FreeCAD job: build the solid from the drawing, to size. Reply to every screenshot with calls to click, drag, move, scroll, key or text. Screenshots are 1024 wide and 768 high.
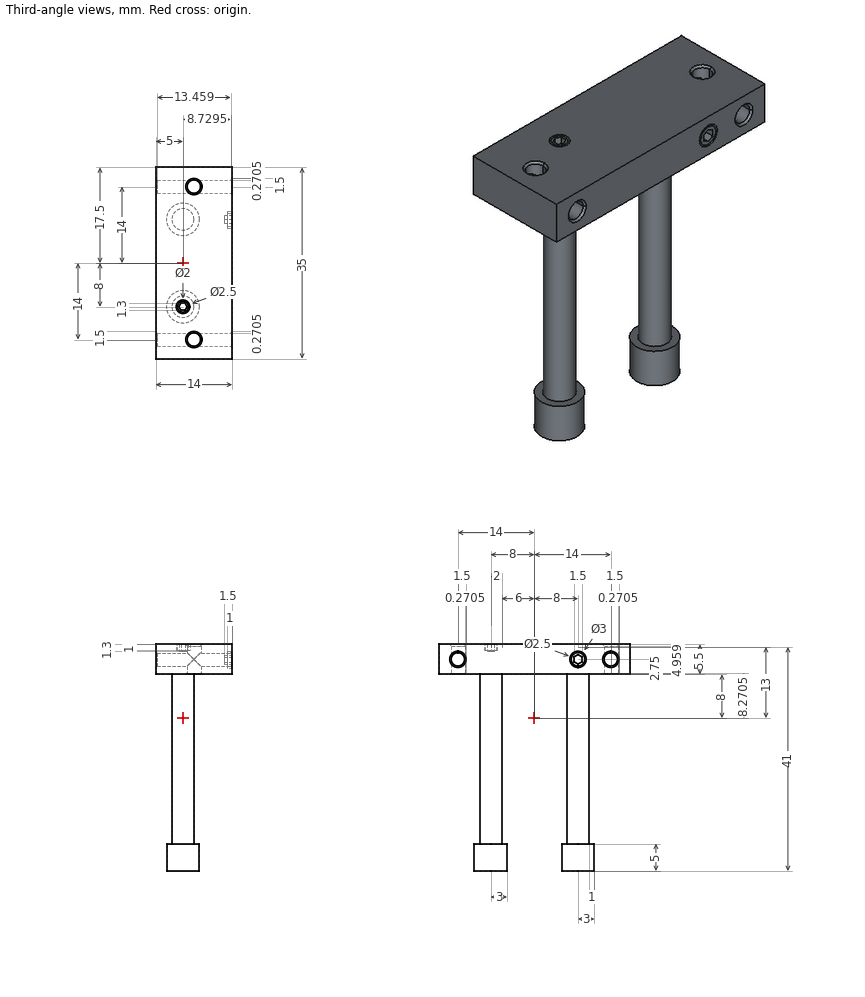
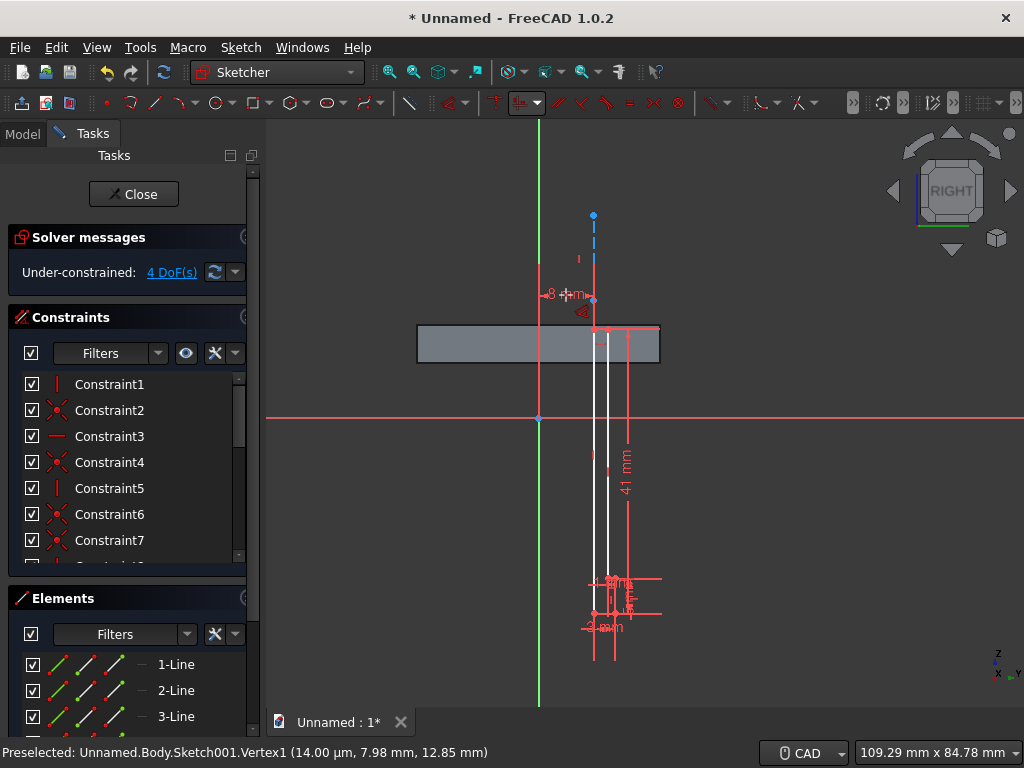
click(594, 301)
click(566, 267)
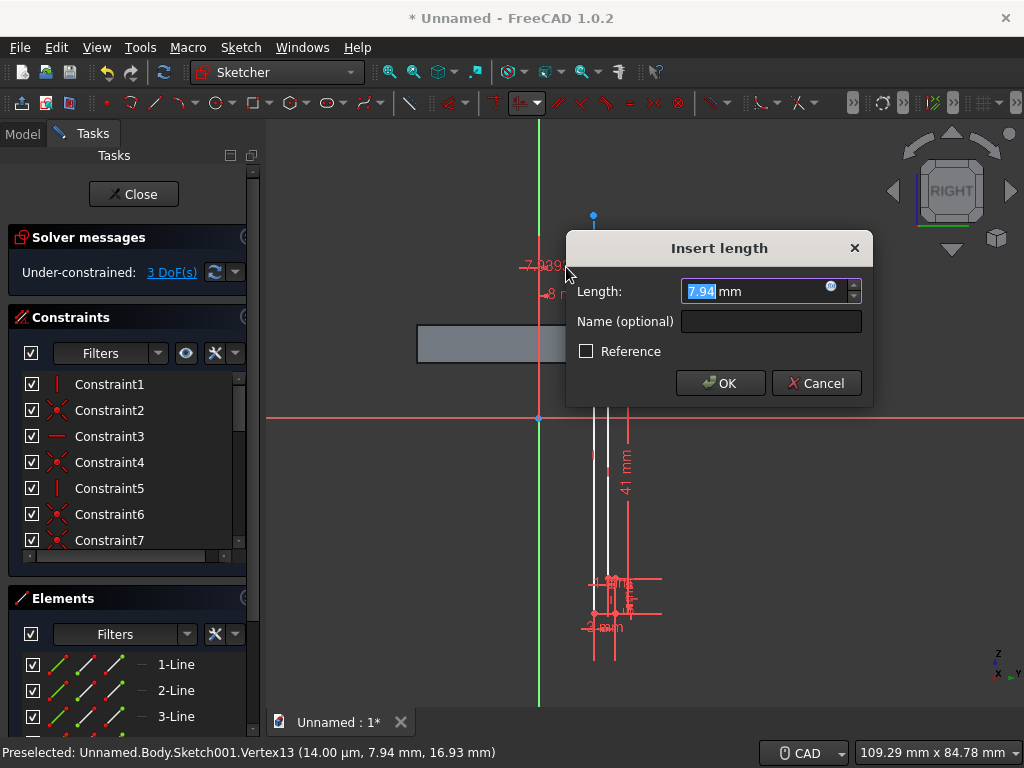
text(8)
key(Return)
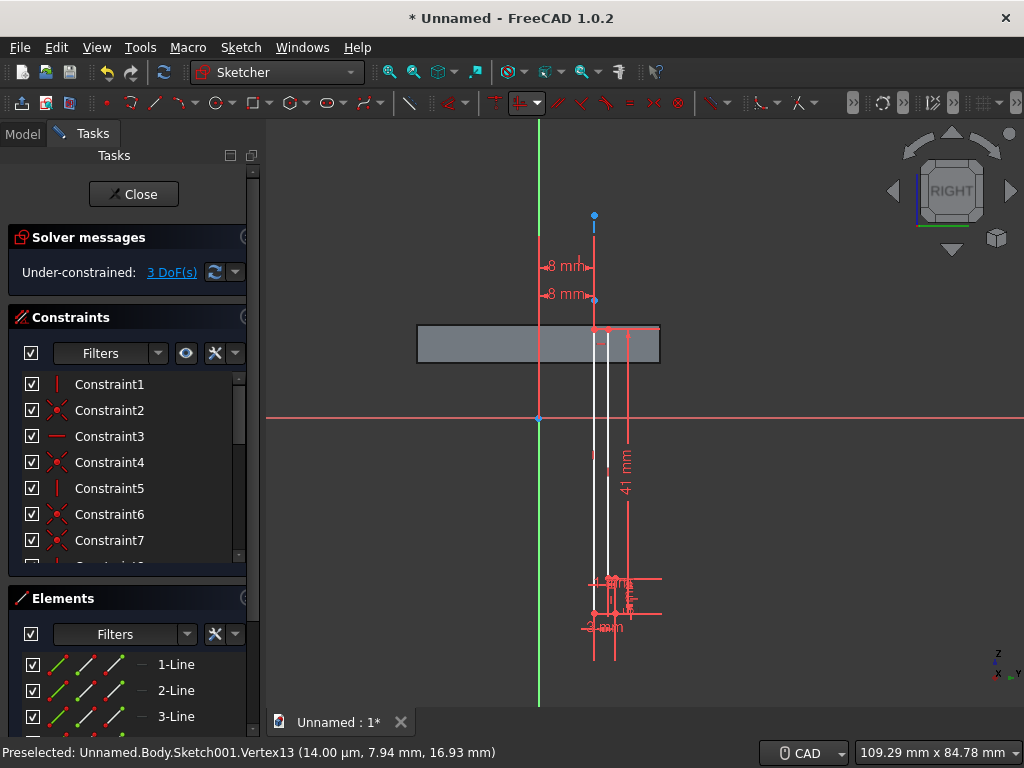
click(594, 329)
click(505, 374)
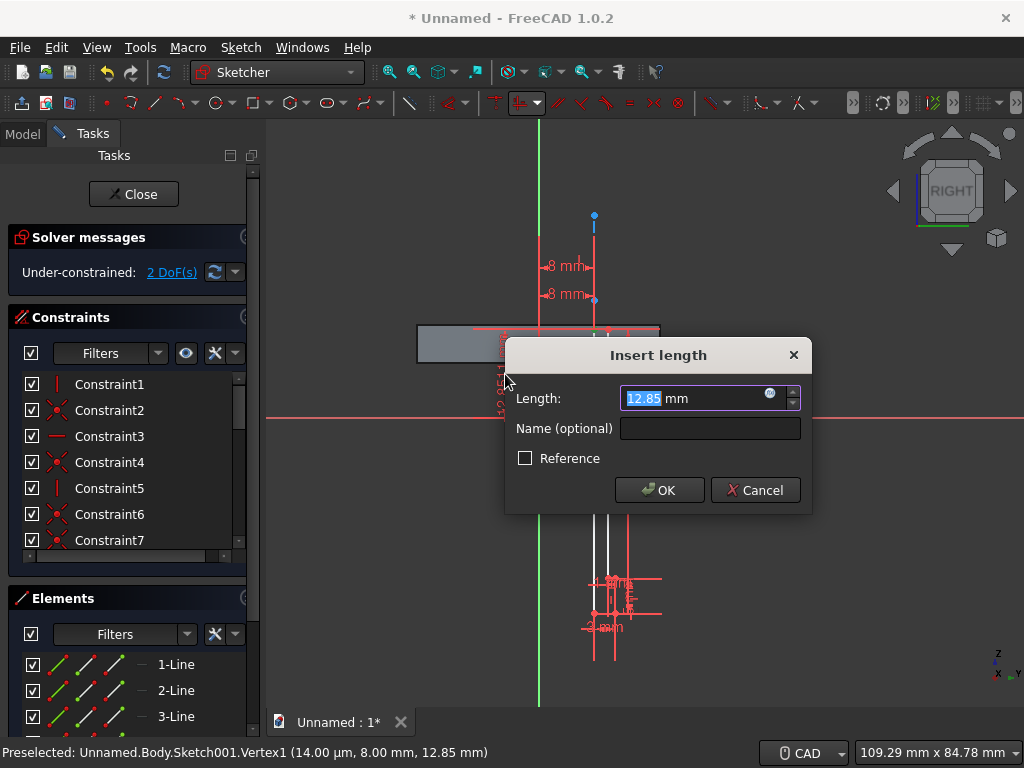
text(13)
key(Return)
key(Escape)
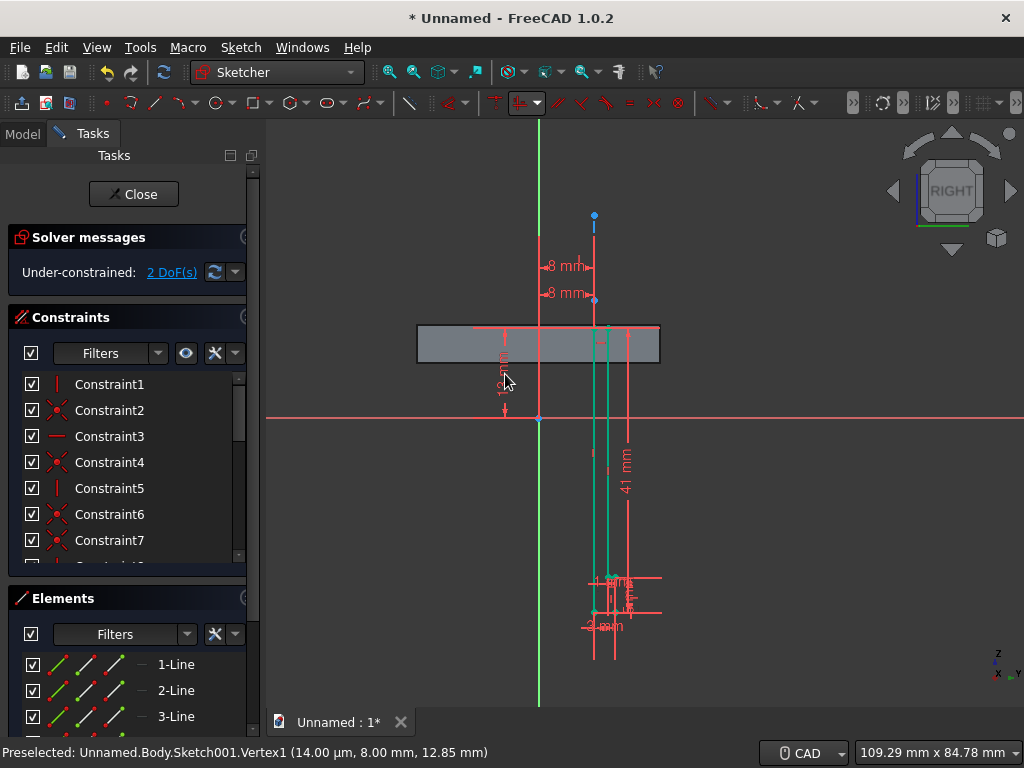
click(134, 194)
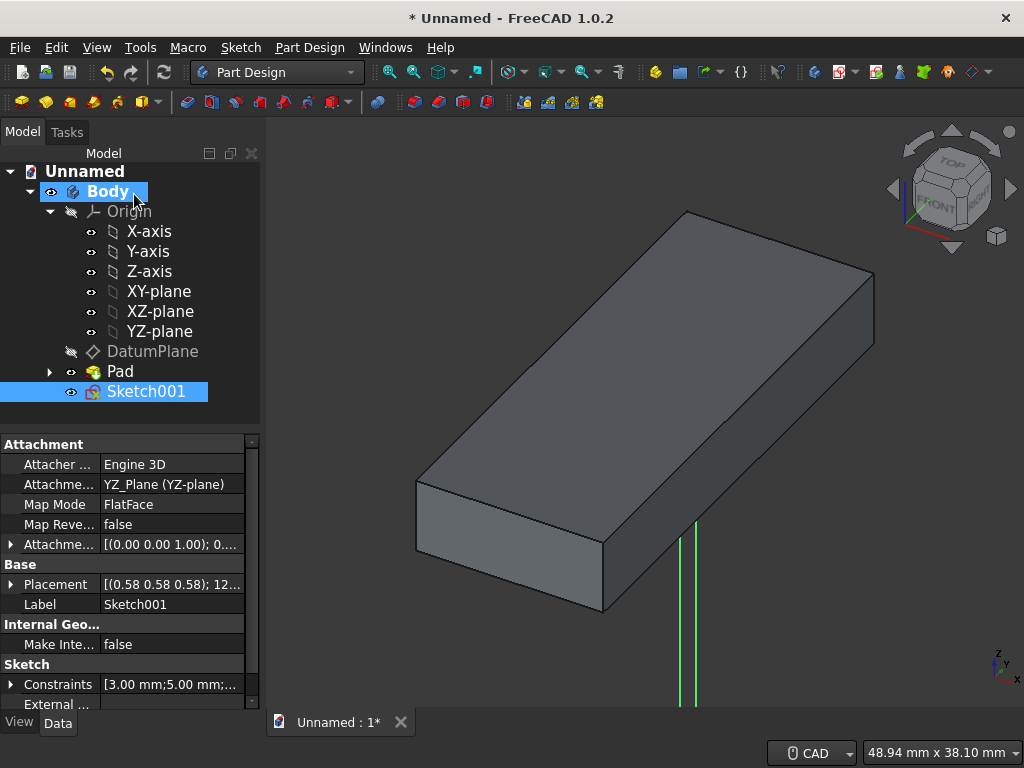
click(46, 102)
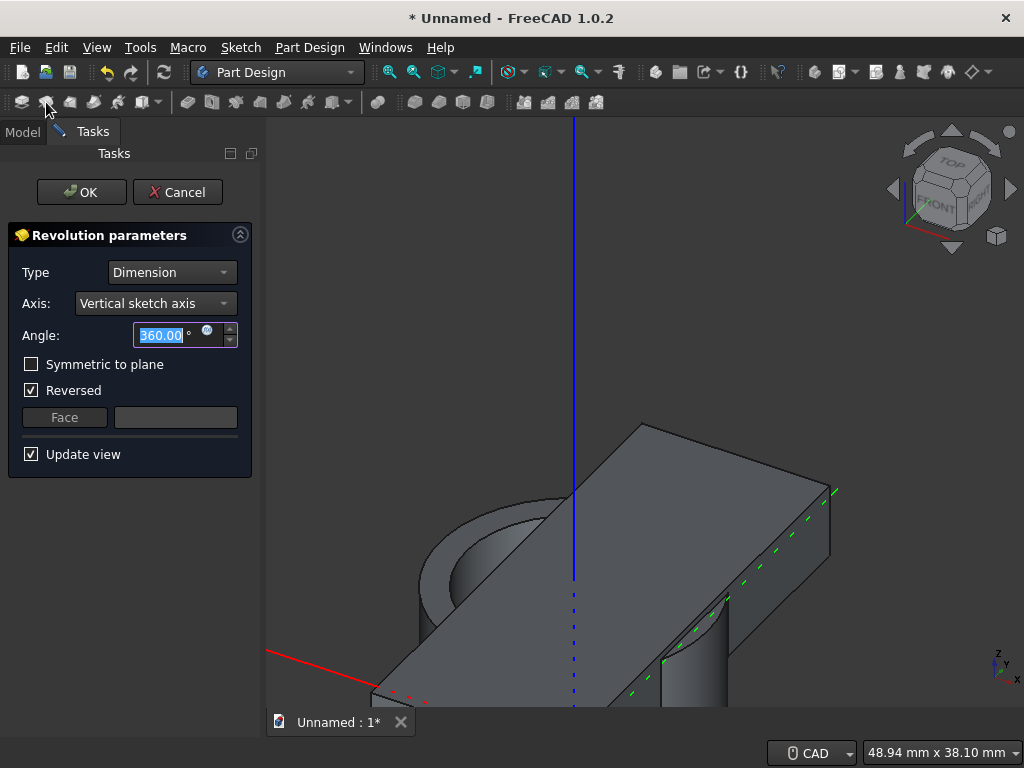
click(156, 304)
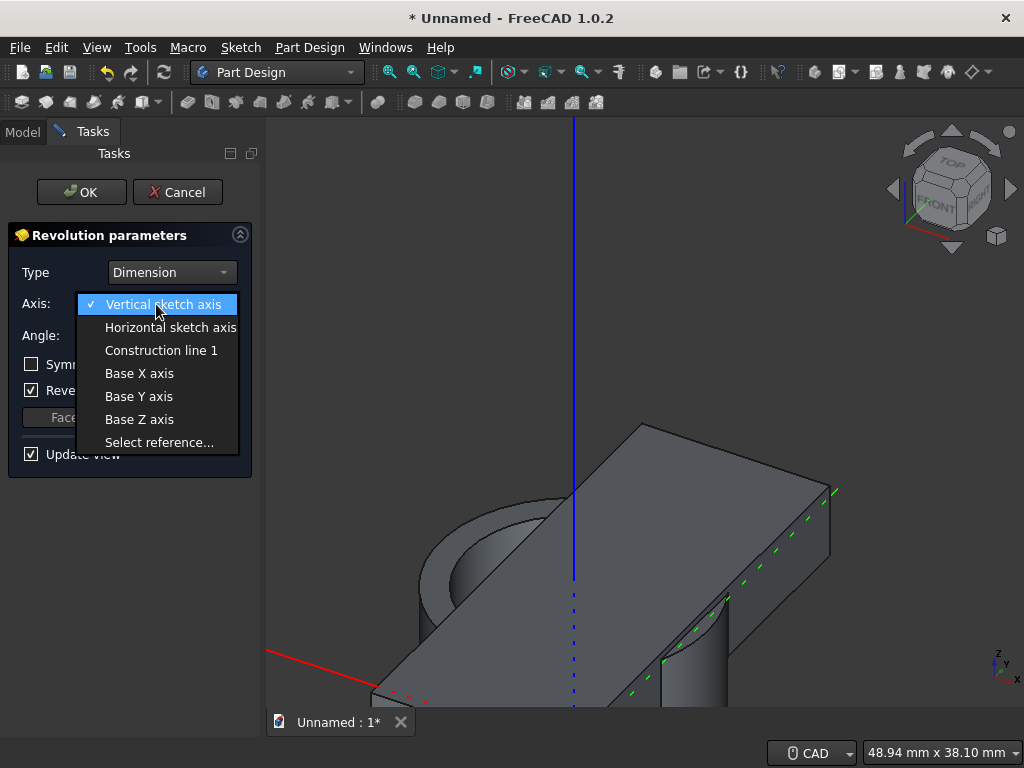
click(156, 350)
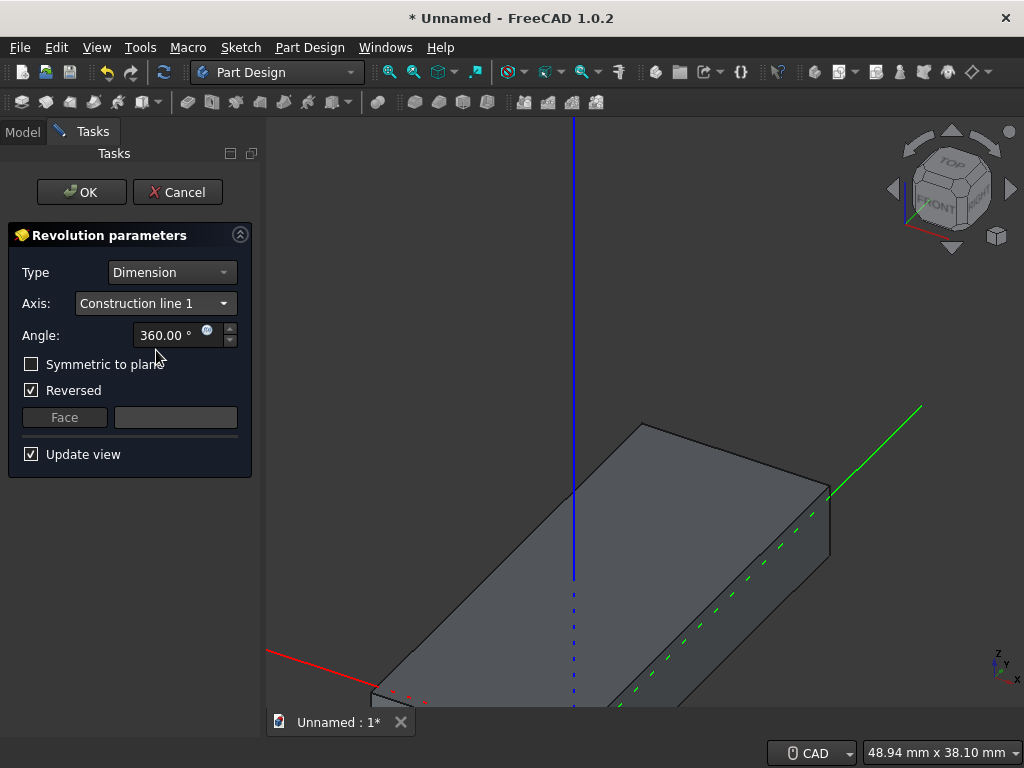
click(82, 192)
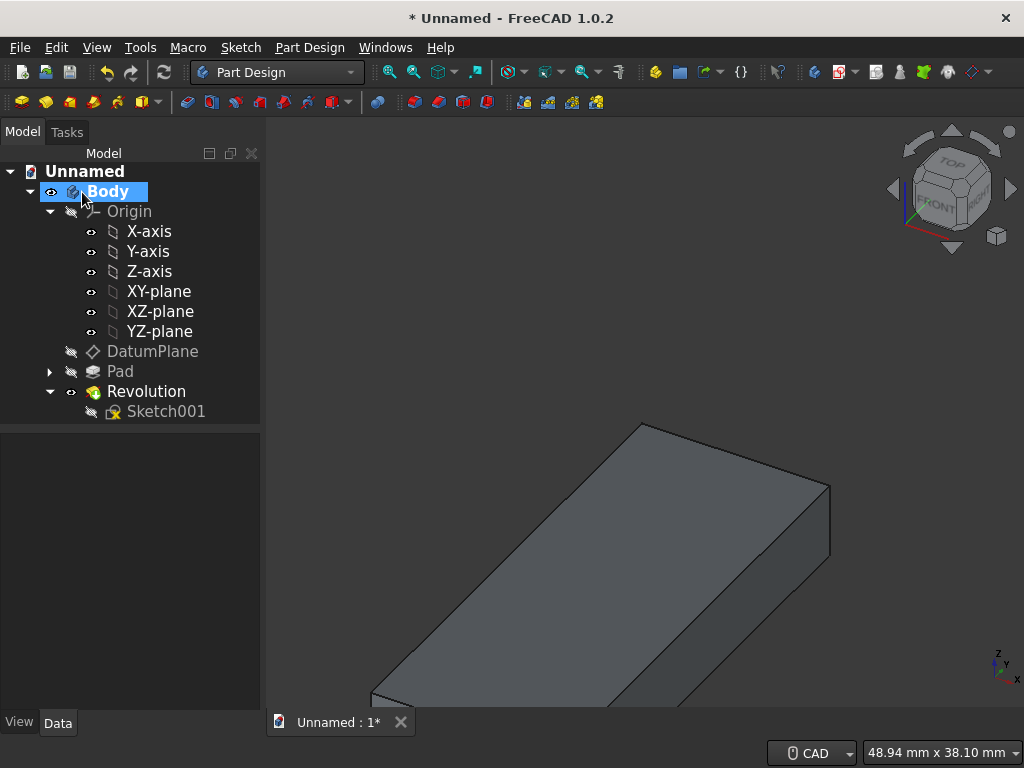
click(390, 72)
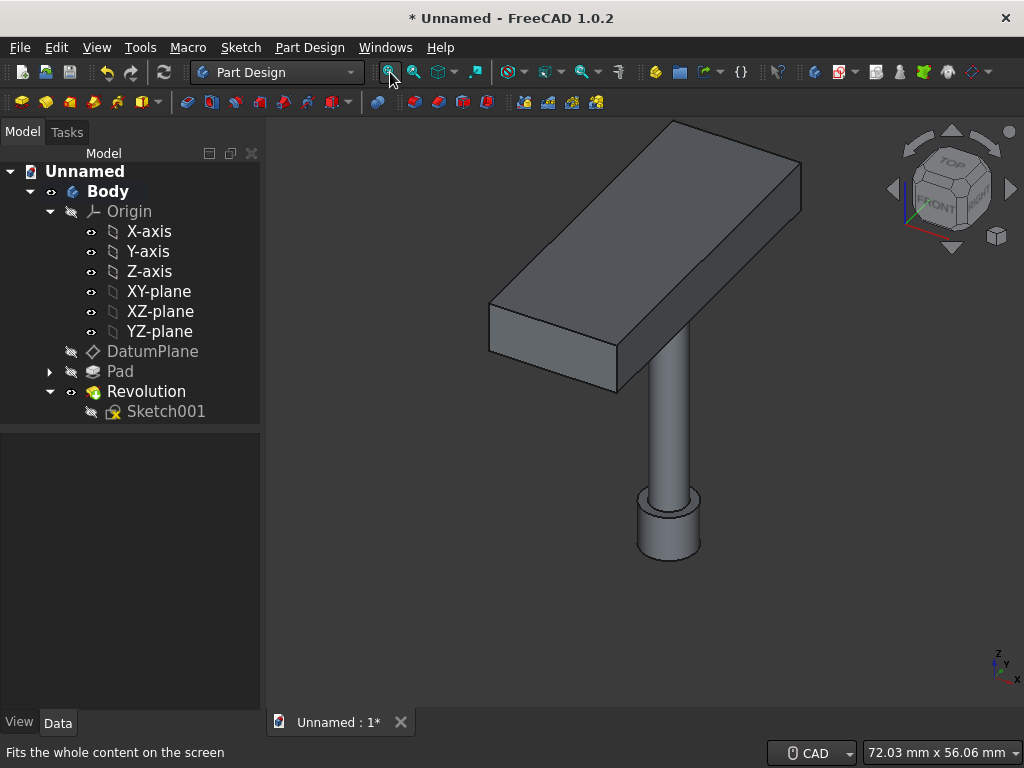
click(840, 72)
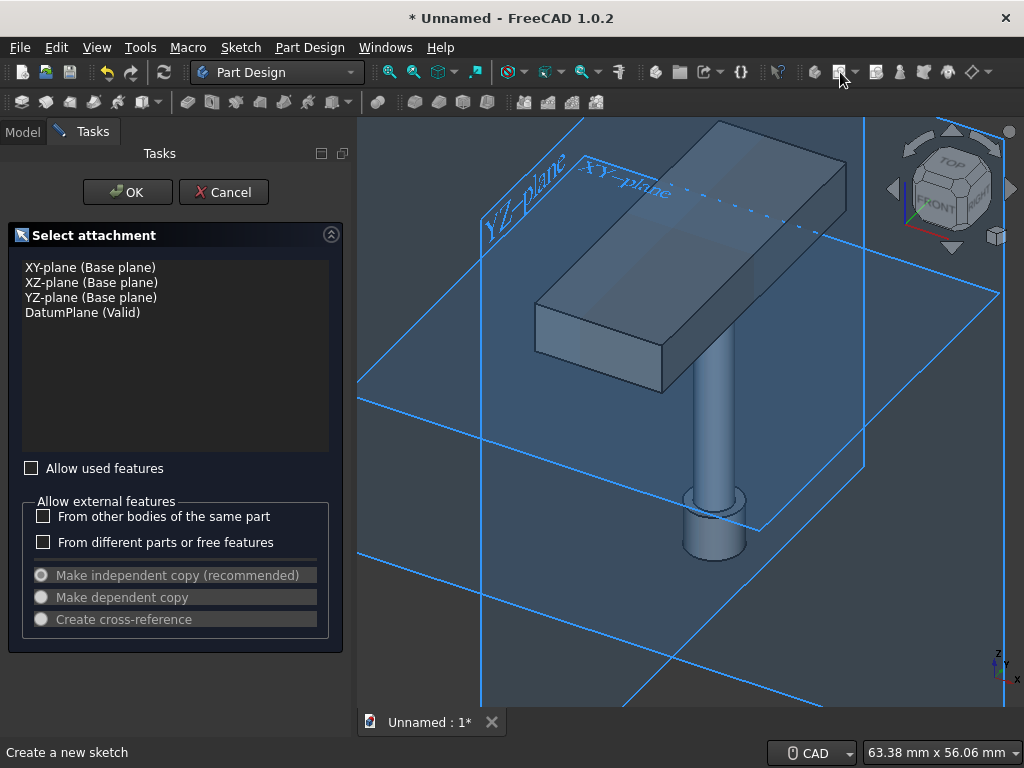
click(82, 298)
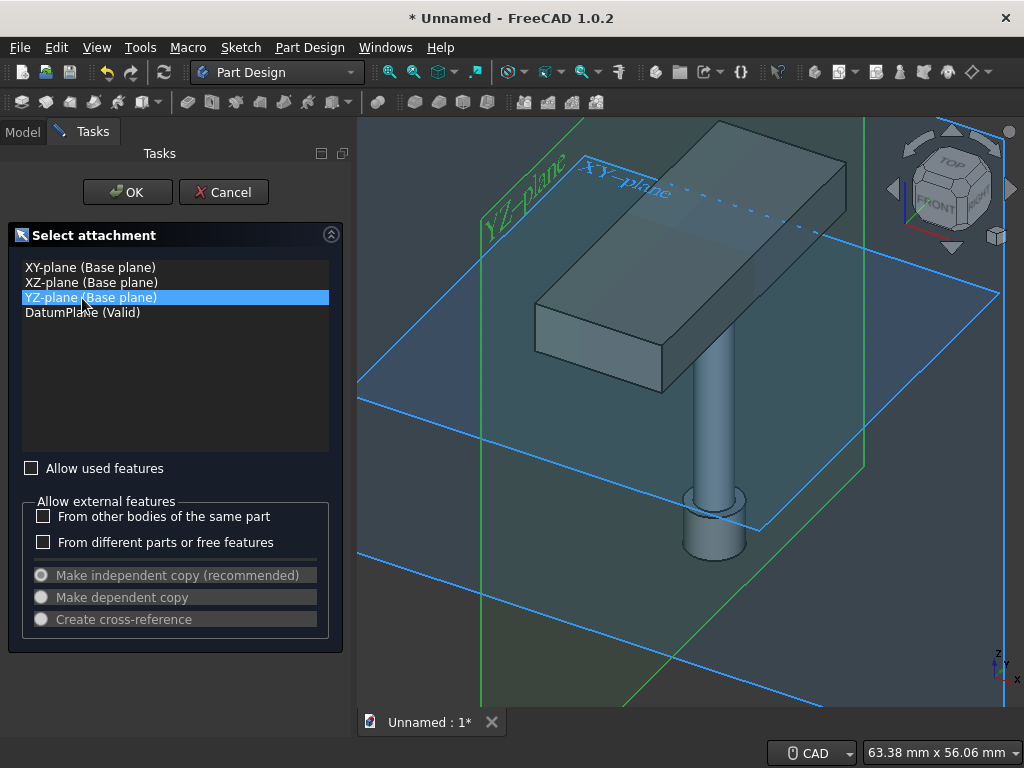
click(128, 192)